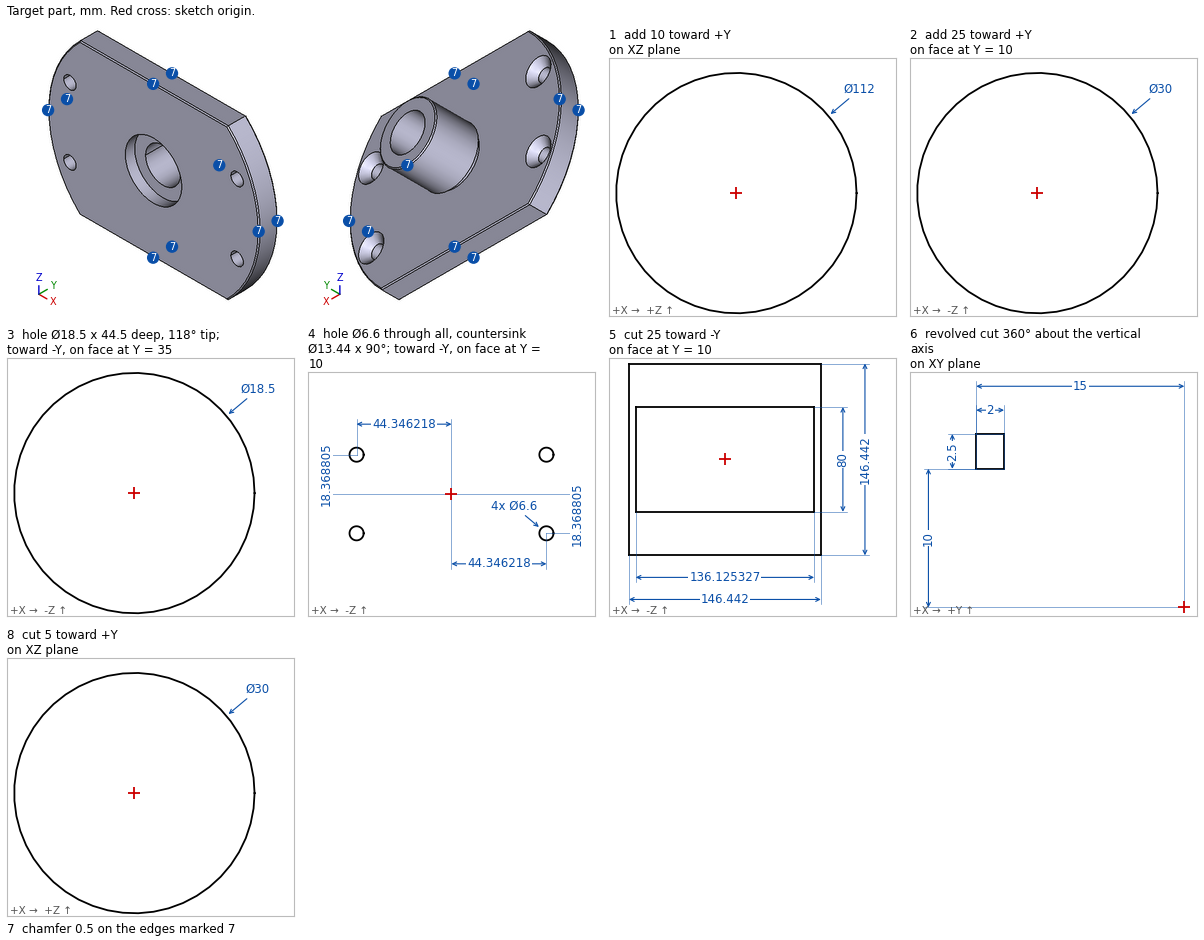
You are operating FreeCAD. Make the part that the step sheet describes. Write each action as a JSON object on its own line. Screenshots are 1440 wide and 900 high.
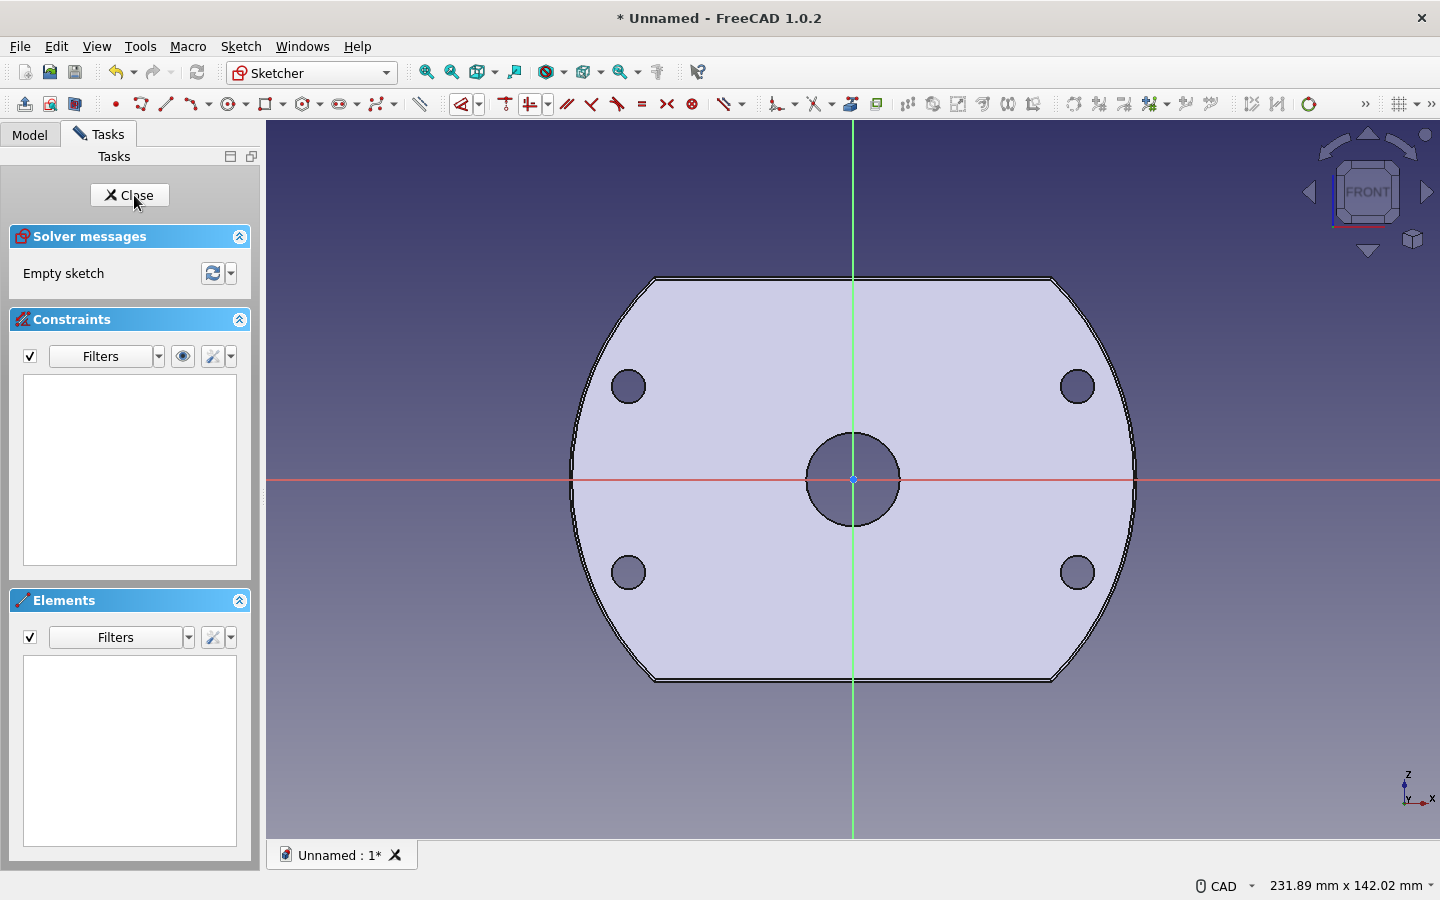
{"action": "scroll", "coordinate": [883, 479], "scroll_direction": "up", "scroll_amount": 6}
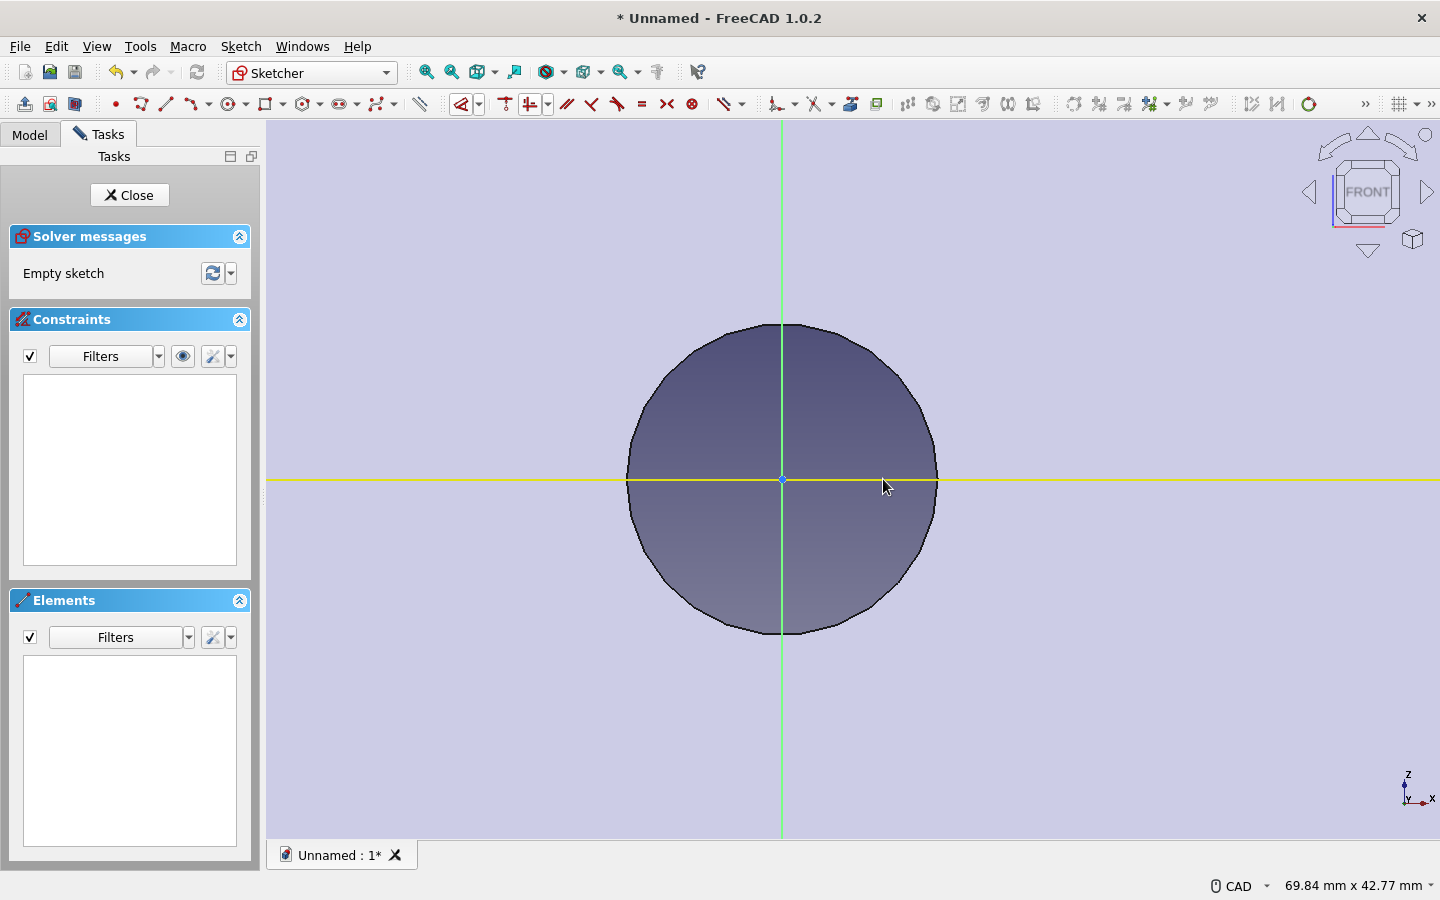
{"action": "left_click", "coordinate": [228, 104]}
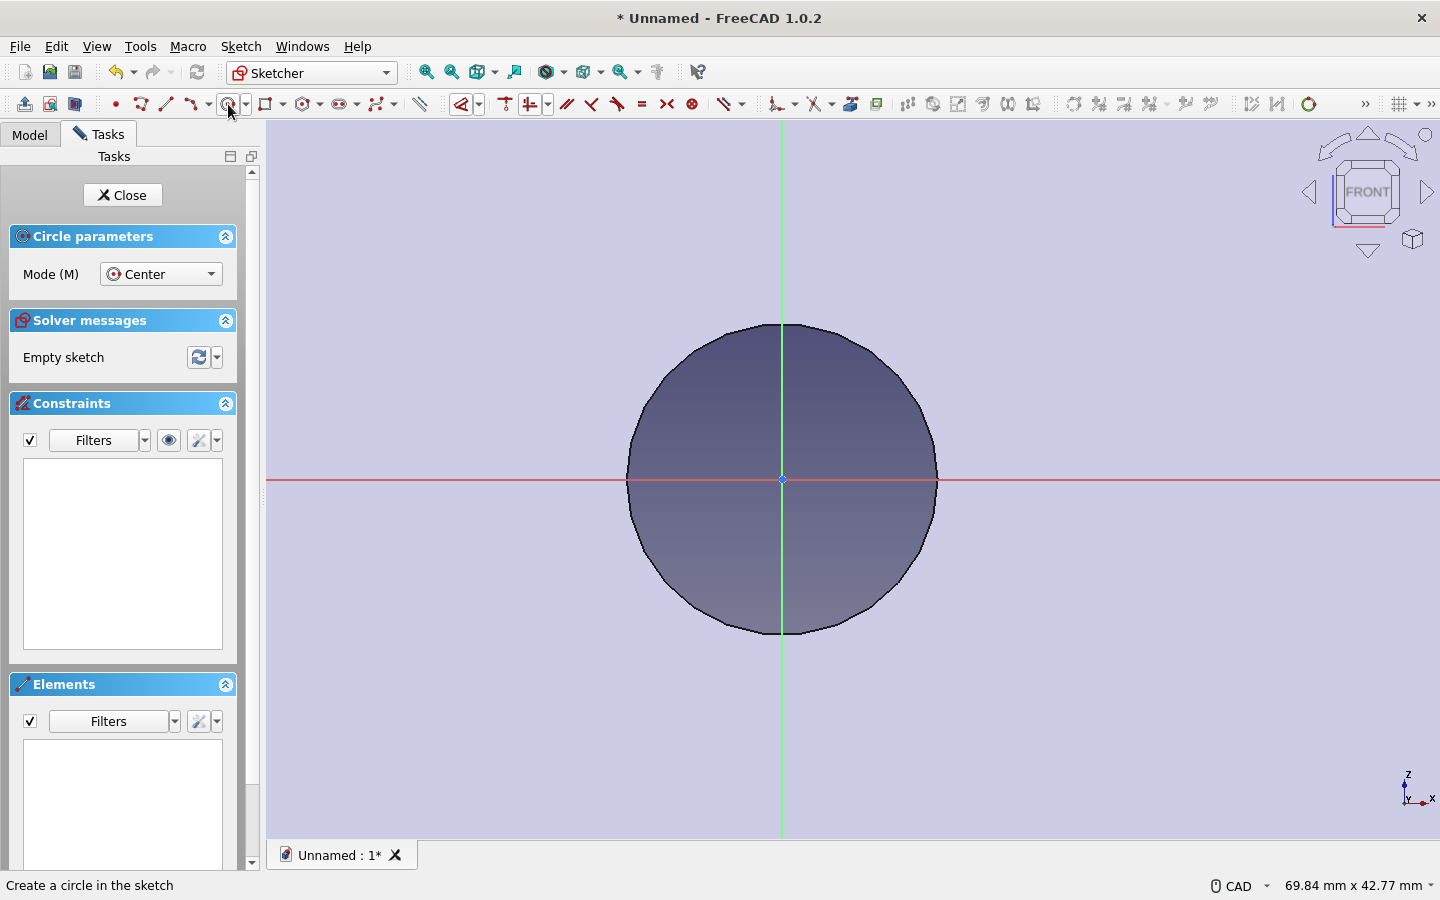
{"action": "left_click", "coordinate": [782, 479]}
{"action": "mouse_move", "coordinate": [960, 301]}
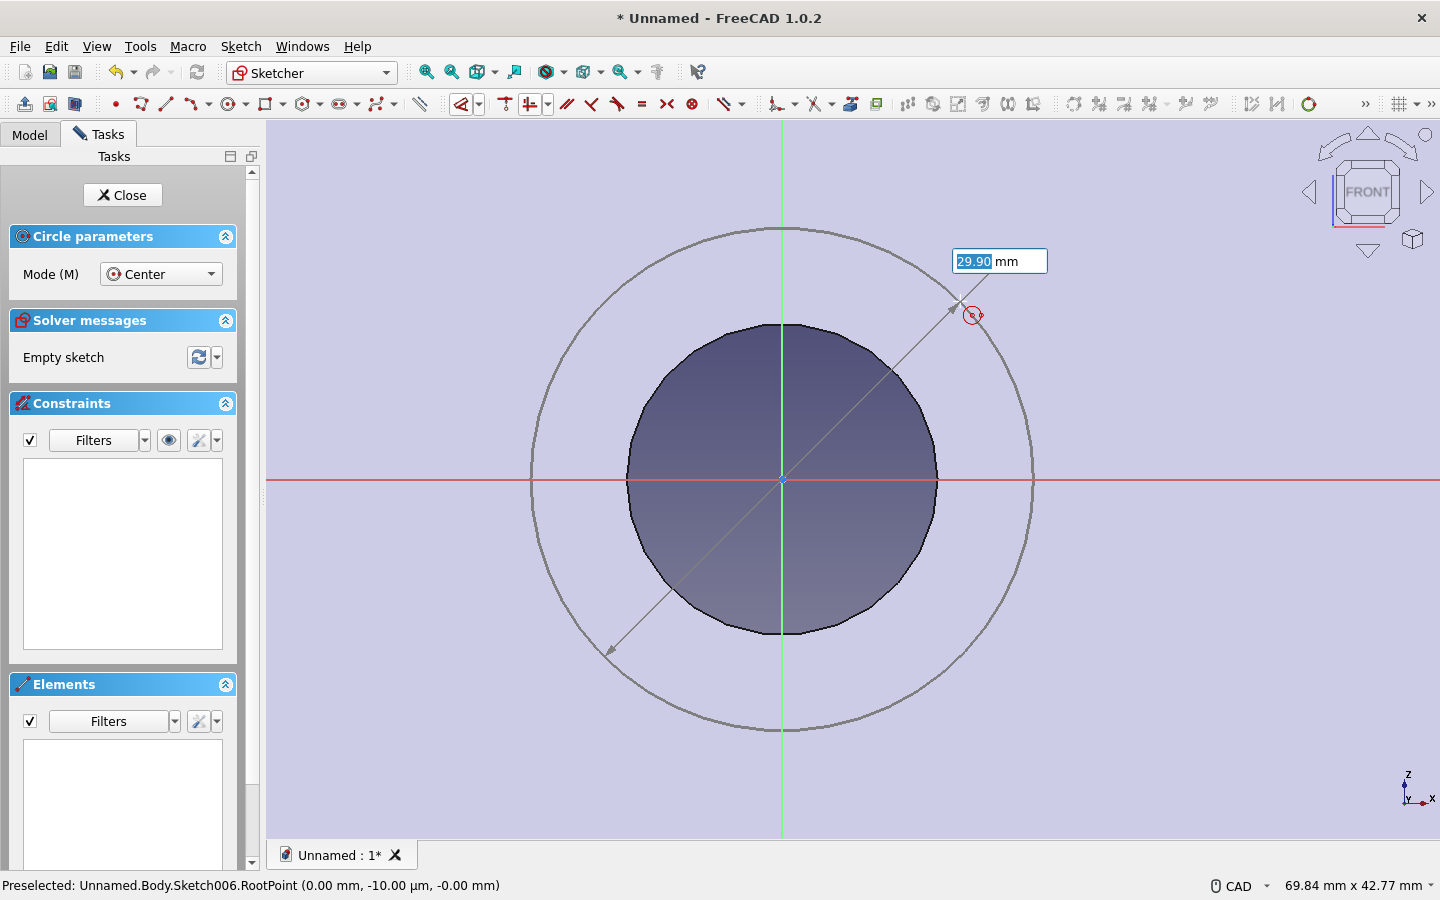
{"action": "type", "text": "30"}
{"action": "key", "text": "Return"}
{"action": "key", "text": "Escape"}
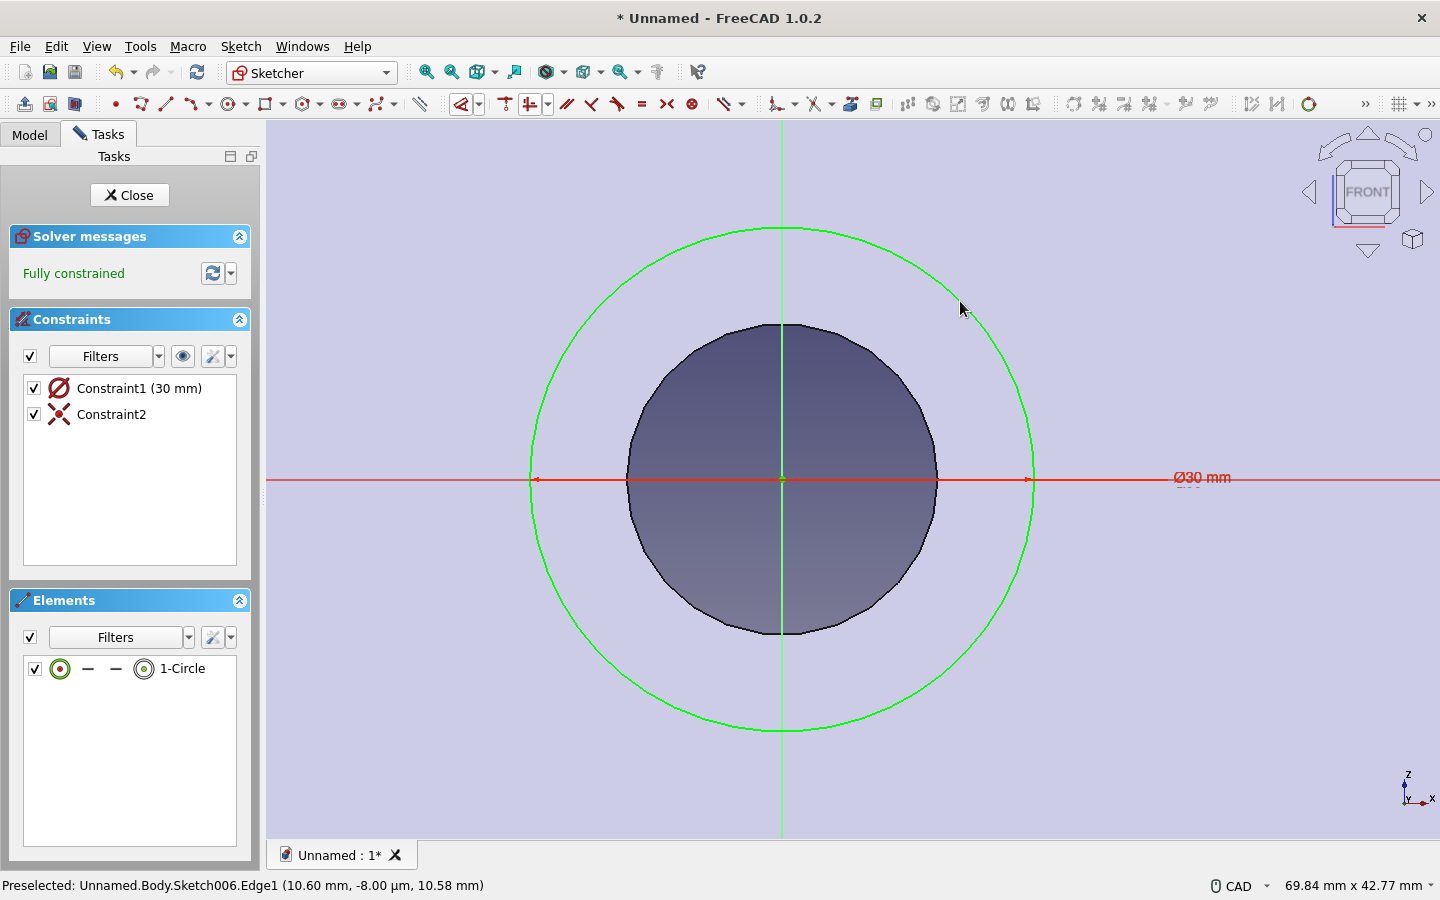
{"action": "left_click", "coordinate": [130, 195]}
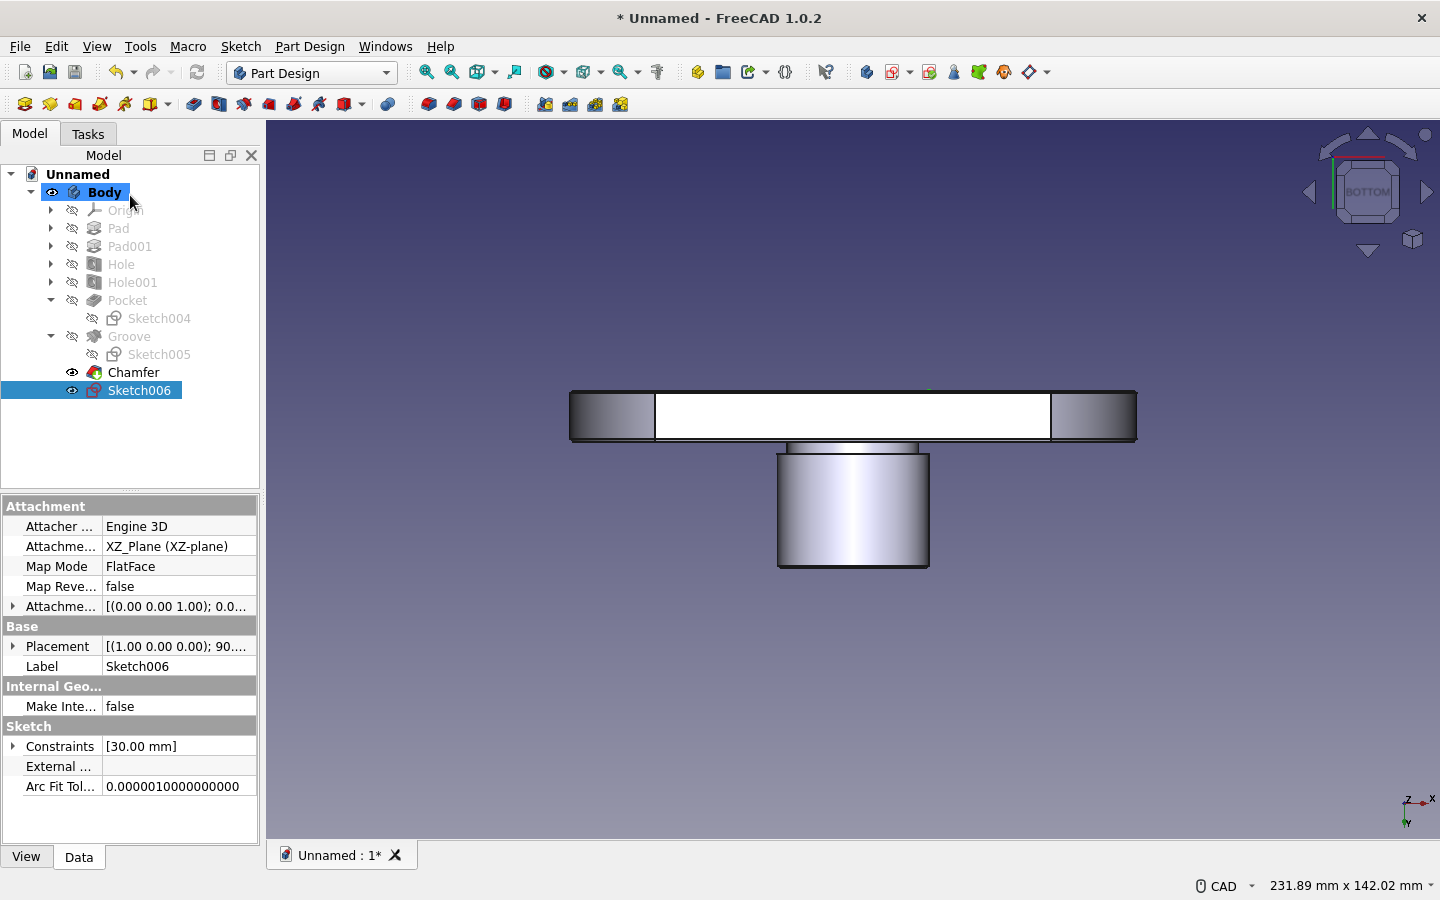
{"action": "left_click", "coordinate": [194, 104]}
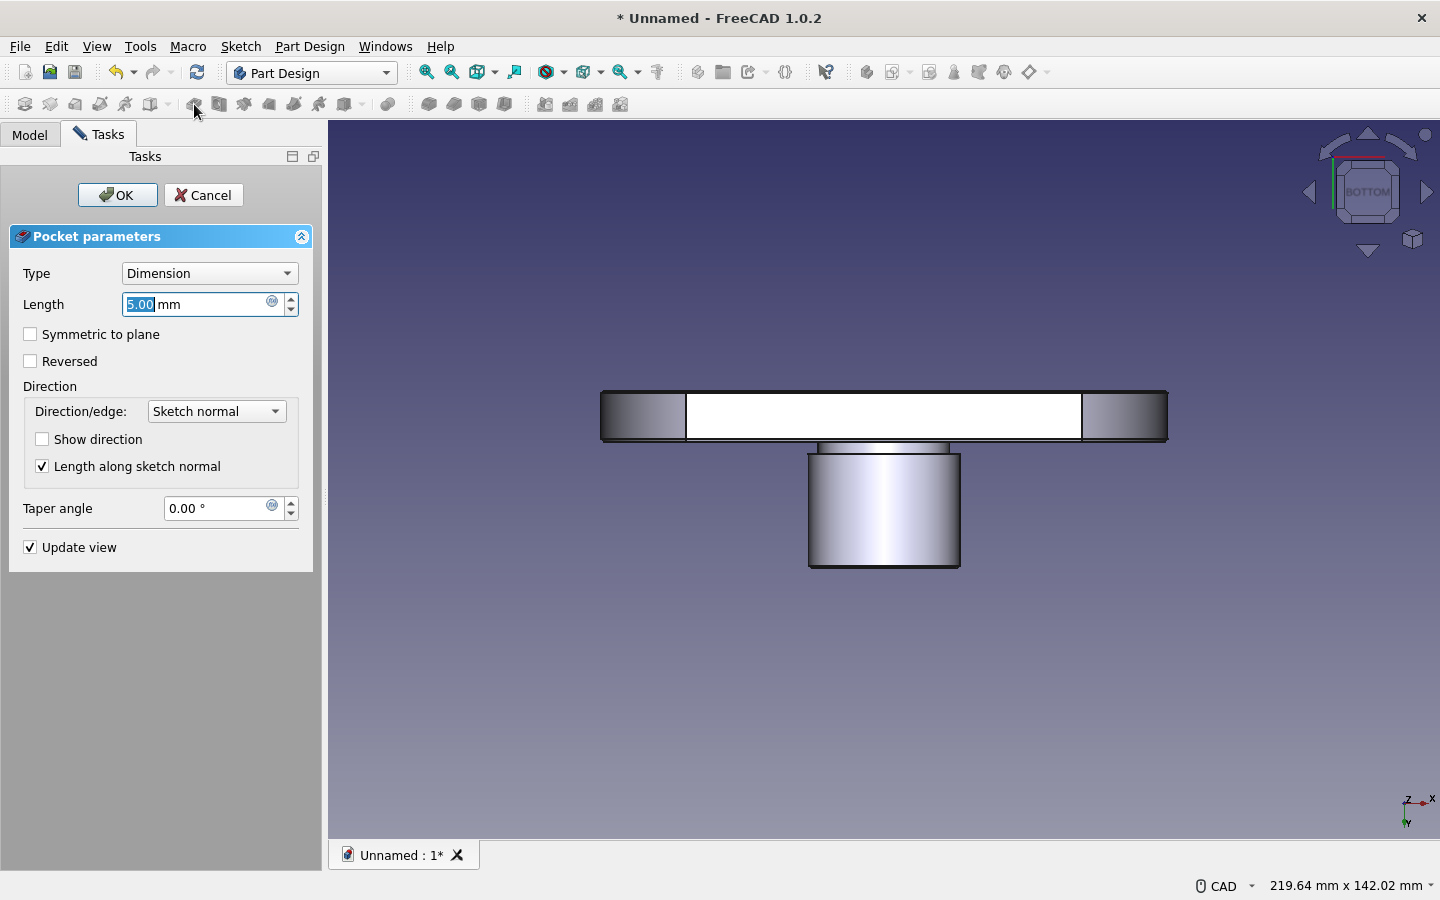
{"action": "type", "text": "5"}
{"action": "key", "text": "Tab"}